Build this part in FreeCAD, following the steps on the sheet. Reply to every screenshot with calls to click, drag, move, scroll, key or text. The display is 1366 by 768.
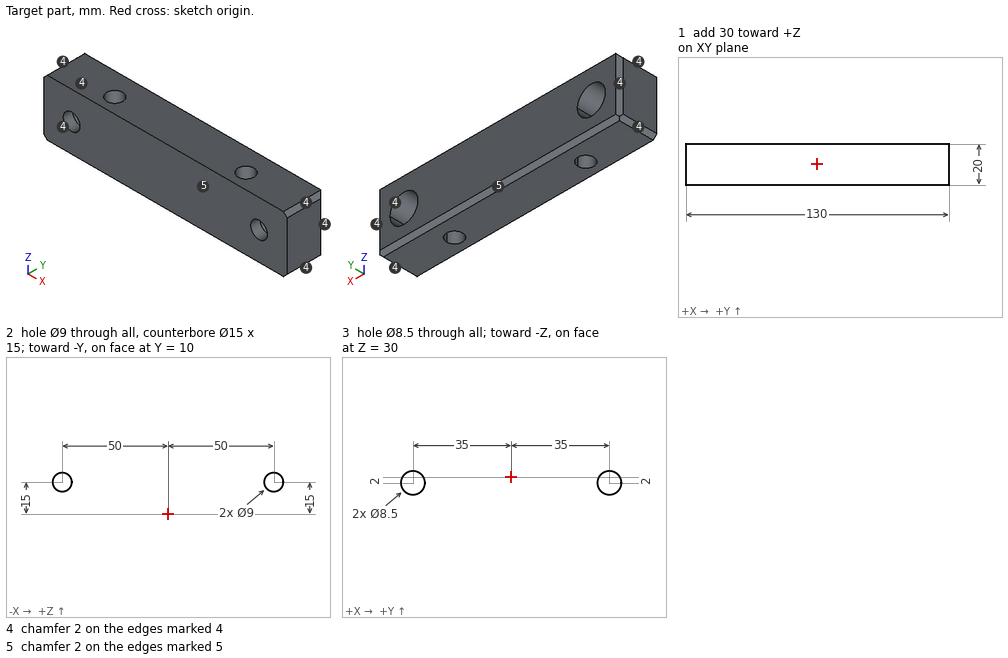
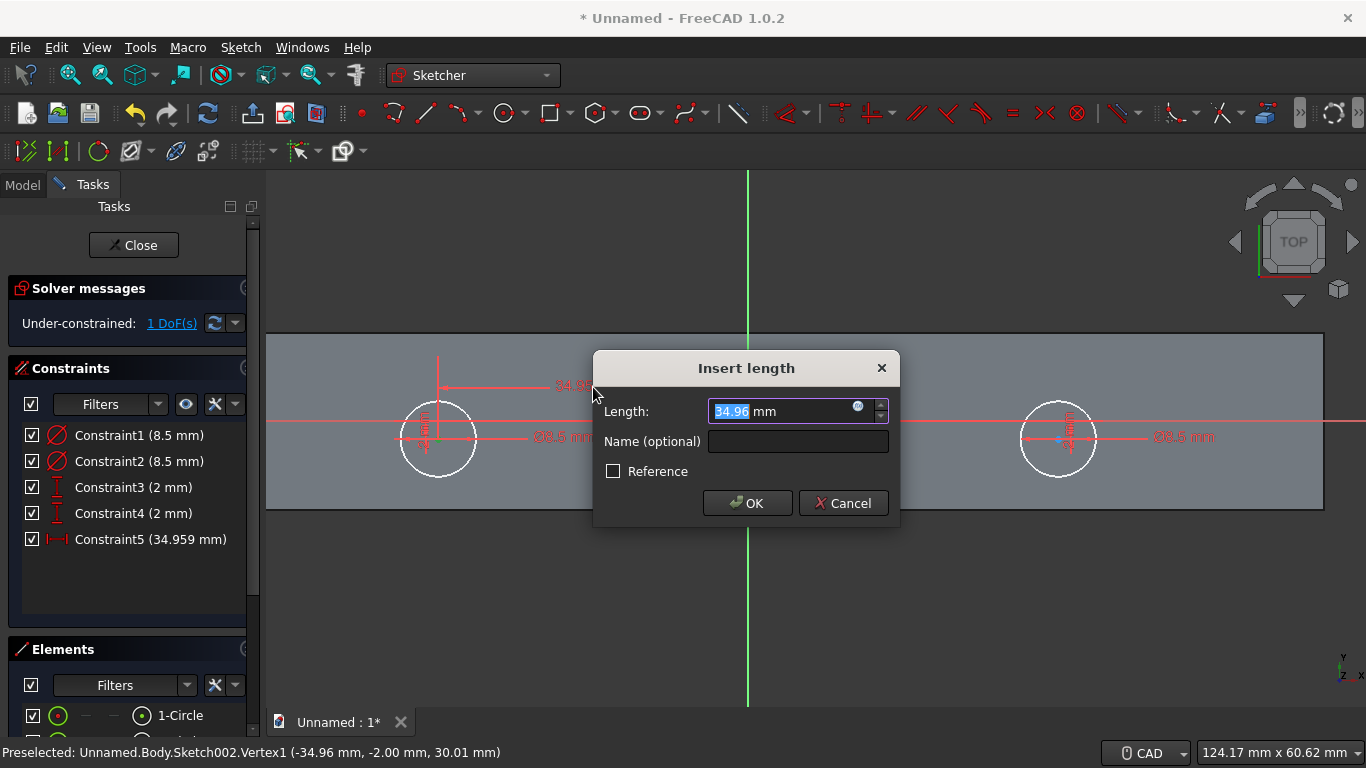
text(35)
key(Return)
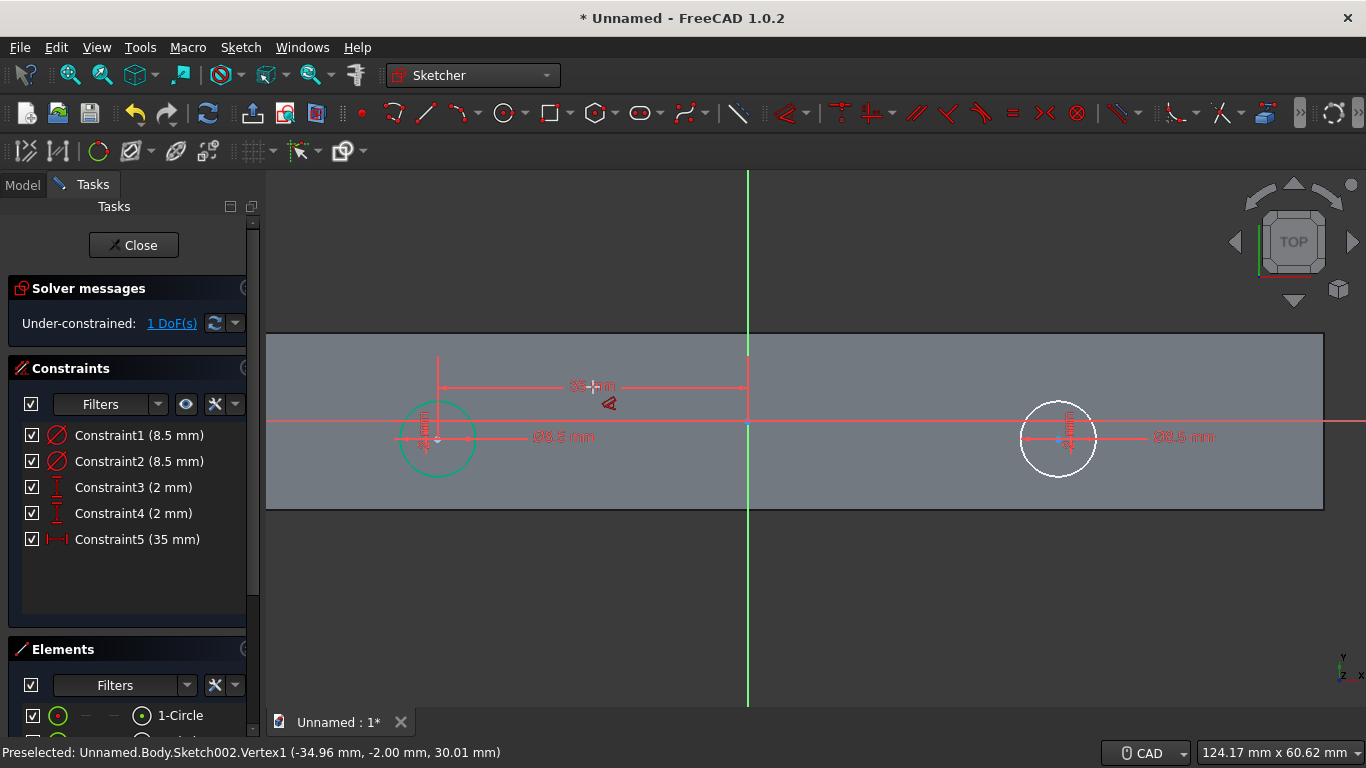
click(1058, 439)
click(903, 387)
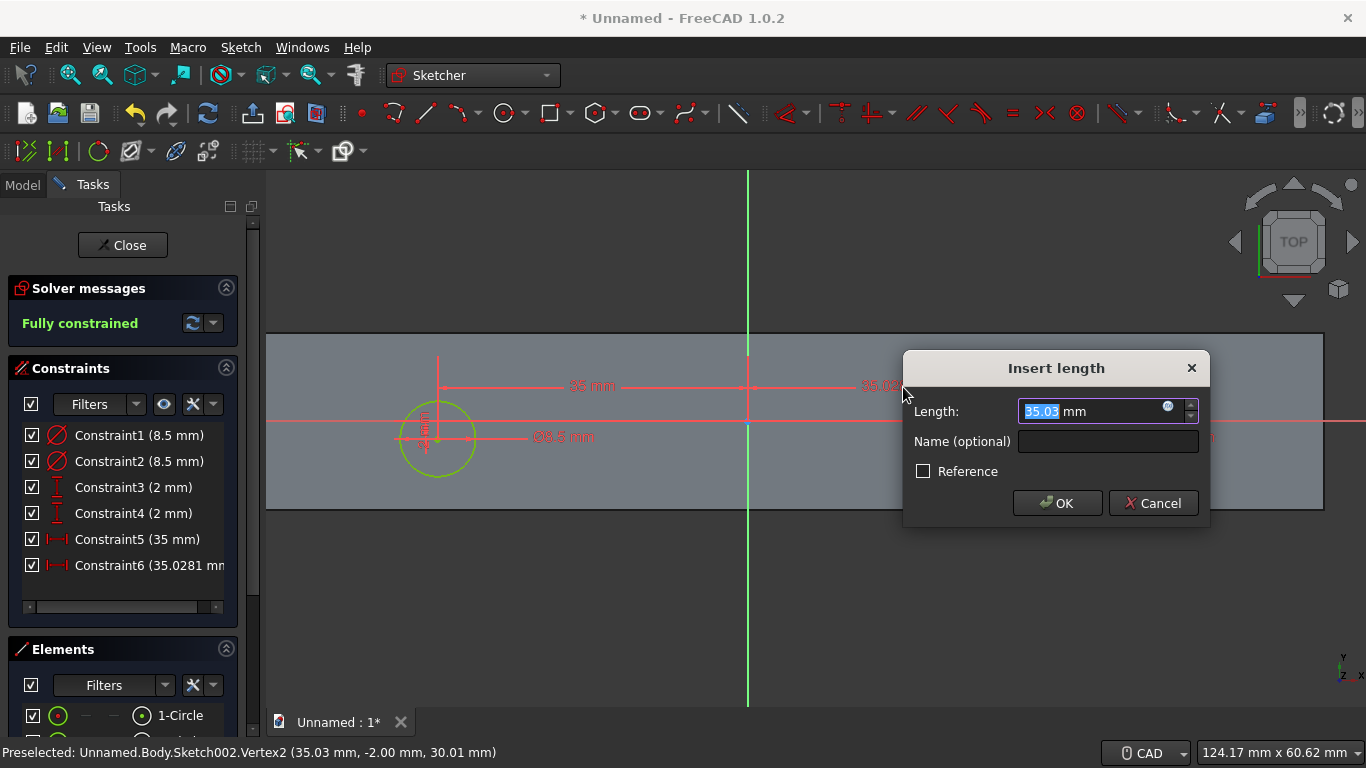
text(35)
key(Return)
key(Escape)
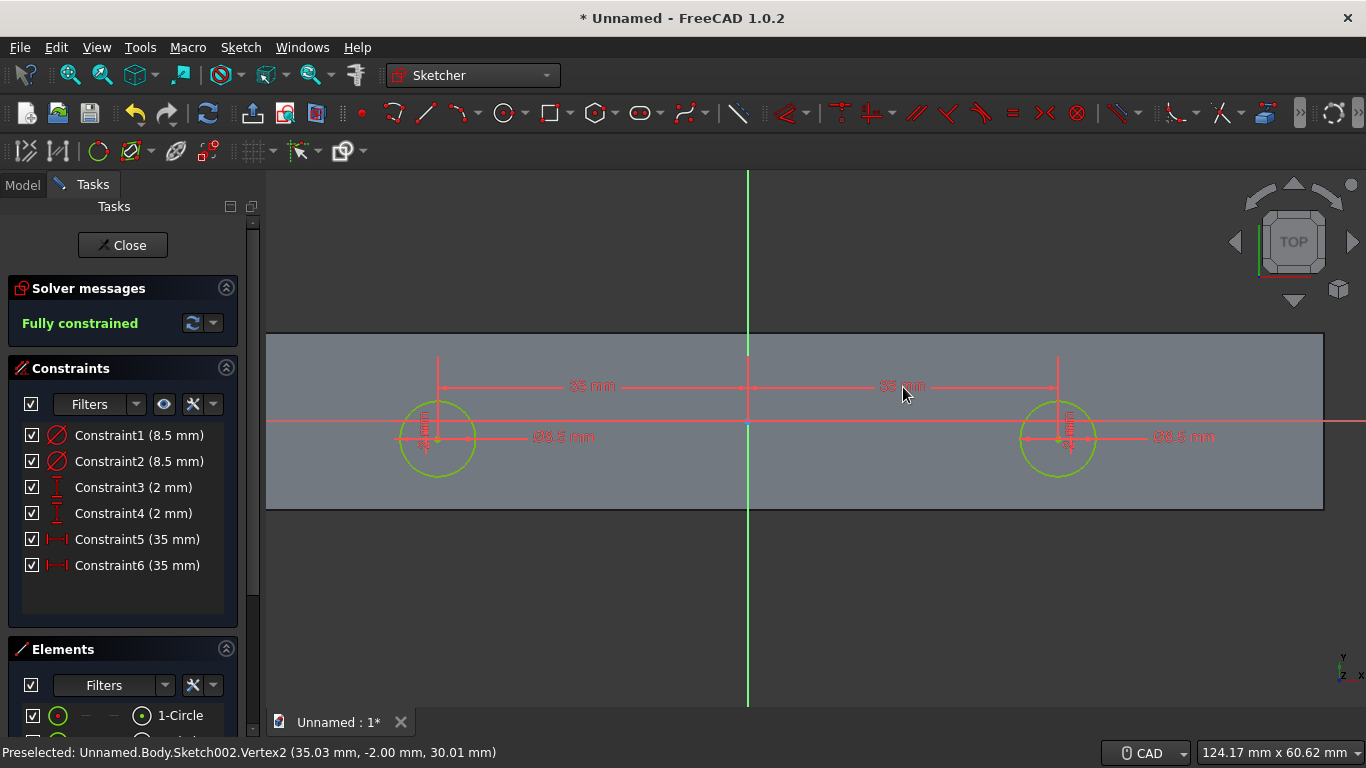
click(123, 245)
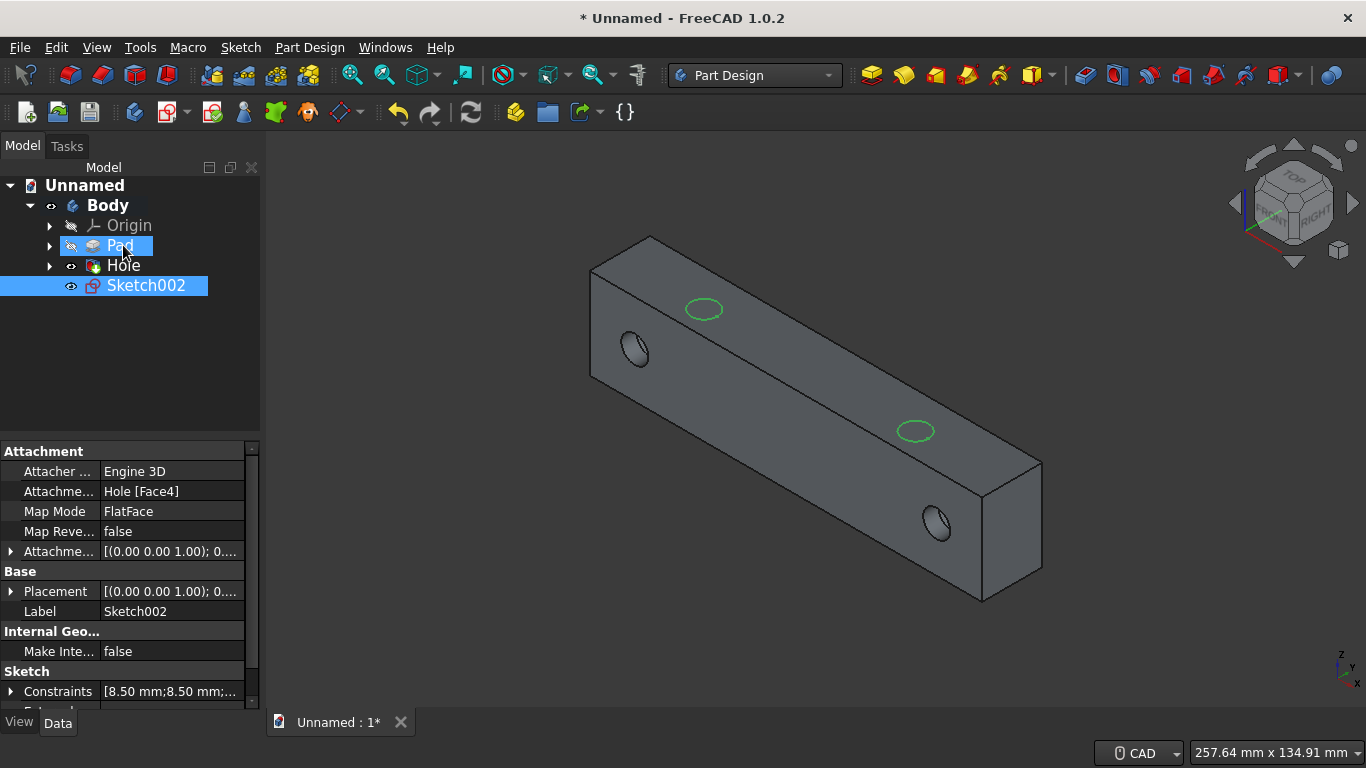
click(1118, 76)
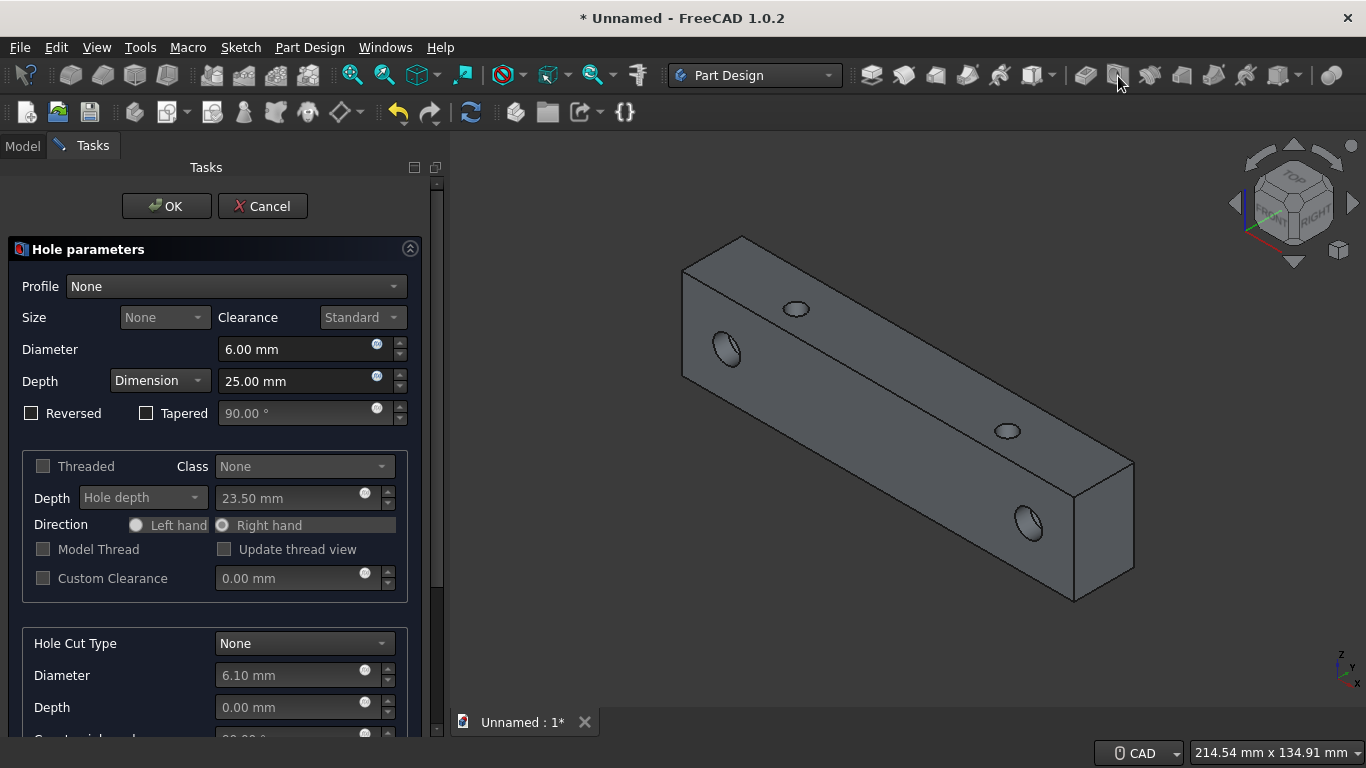
triple_click(305, 349)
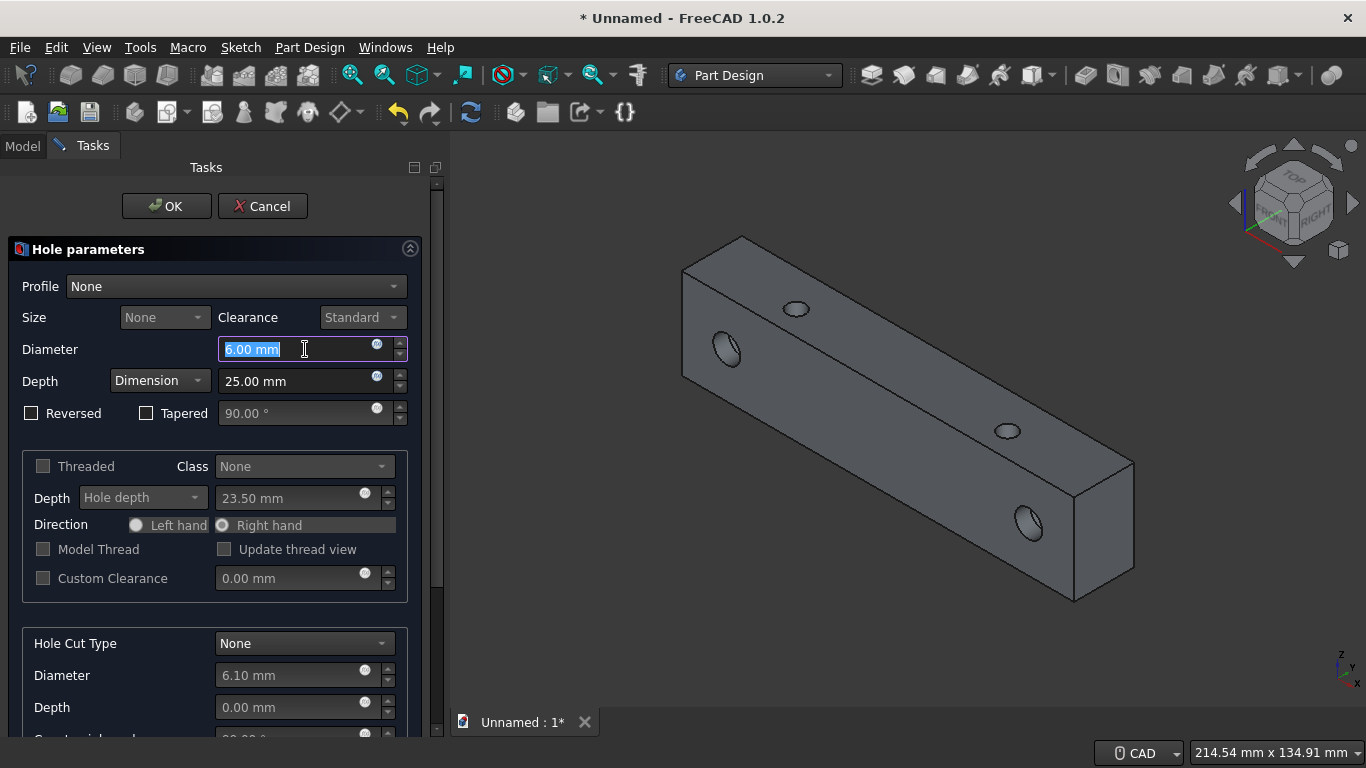
text(8.5)
key(Tab)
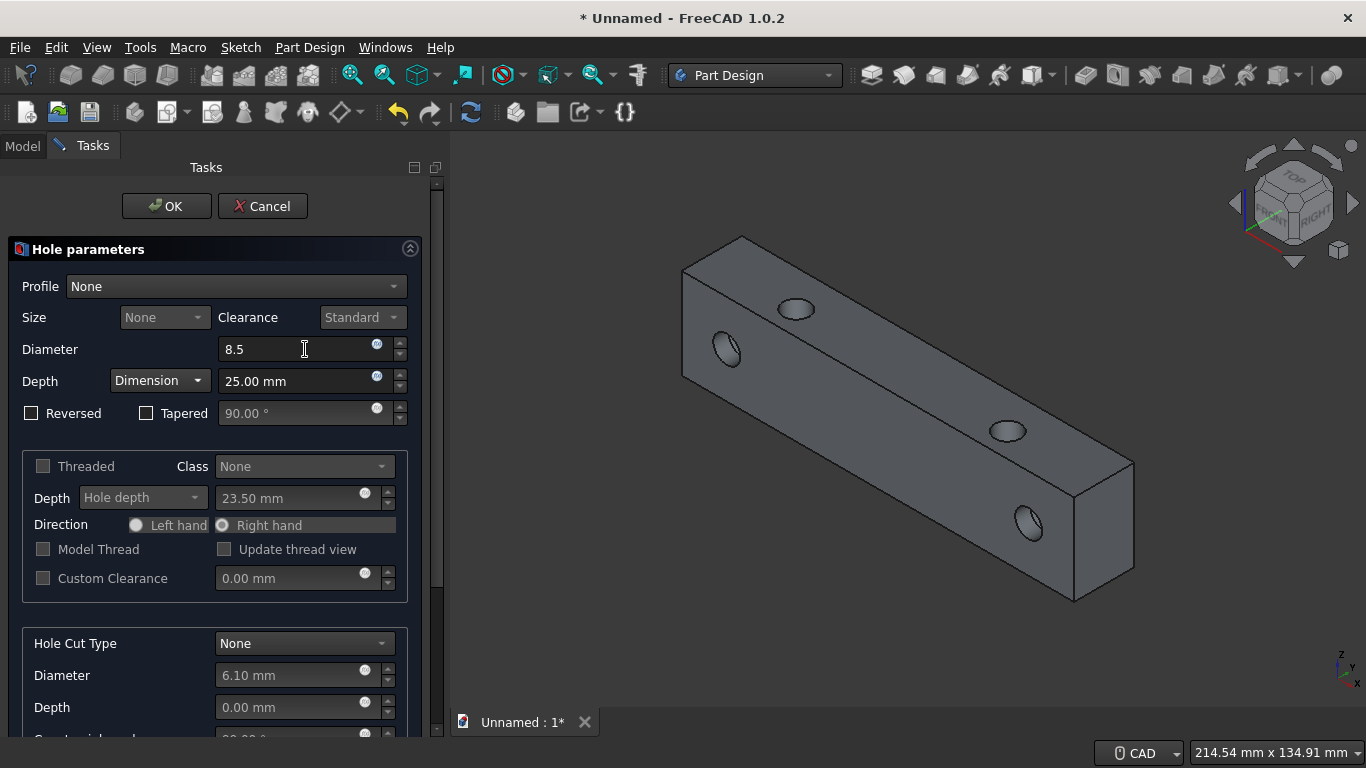
click(161, 380)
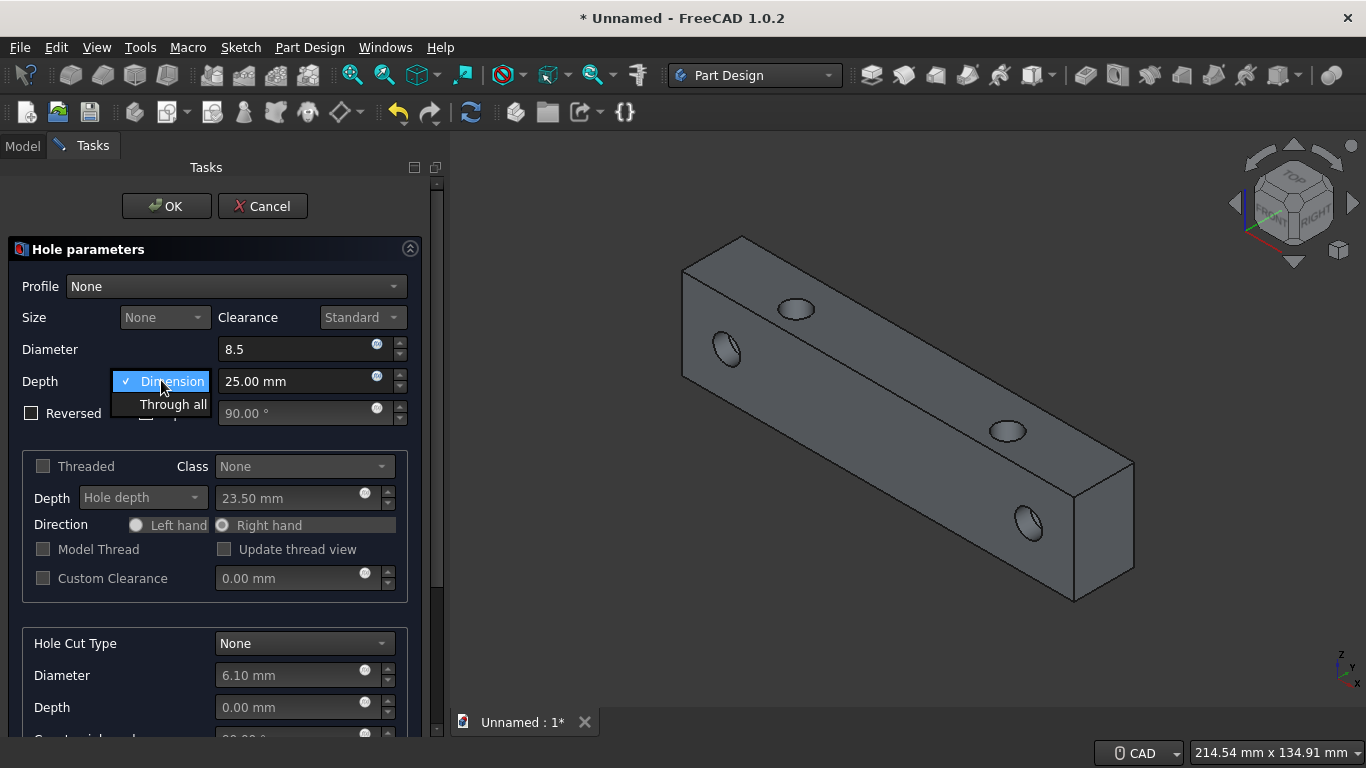
click(160, 404)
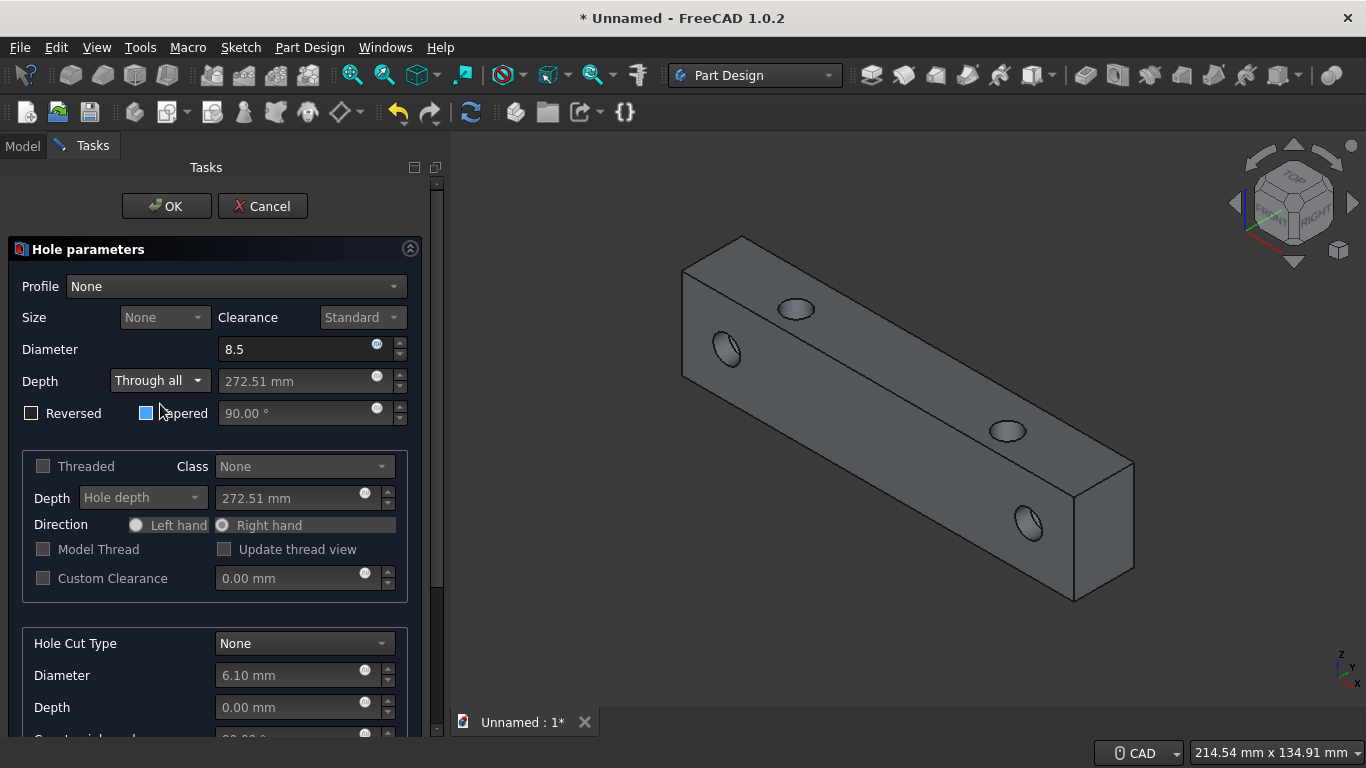
click(167, 206)